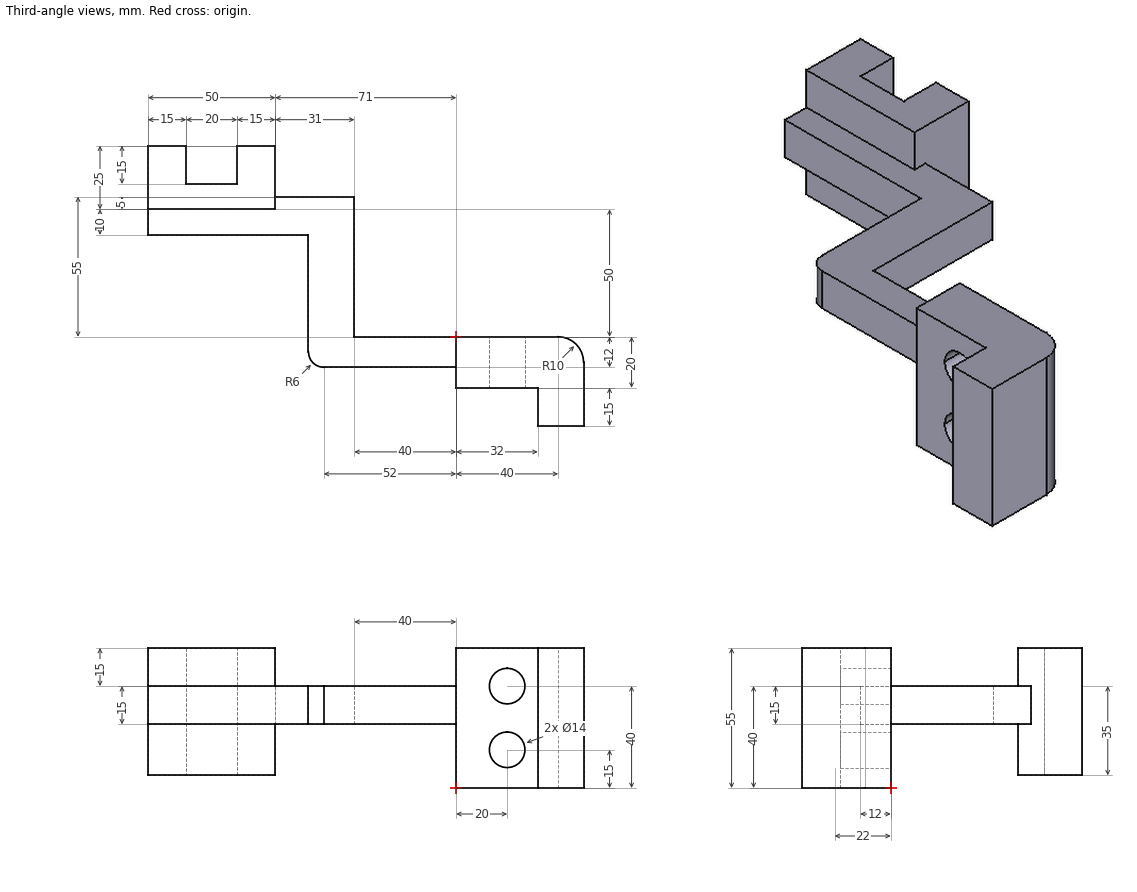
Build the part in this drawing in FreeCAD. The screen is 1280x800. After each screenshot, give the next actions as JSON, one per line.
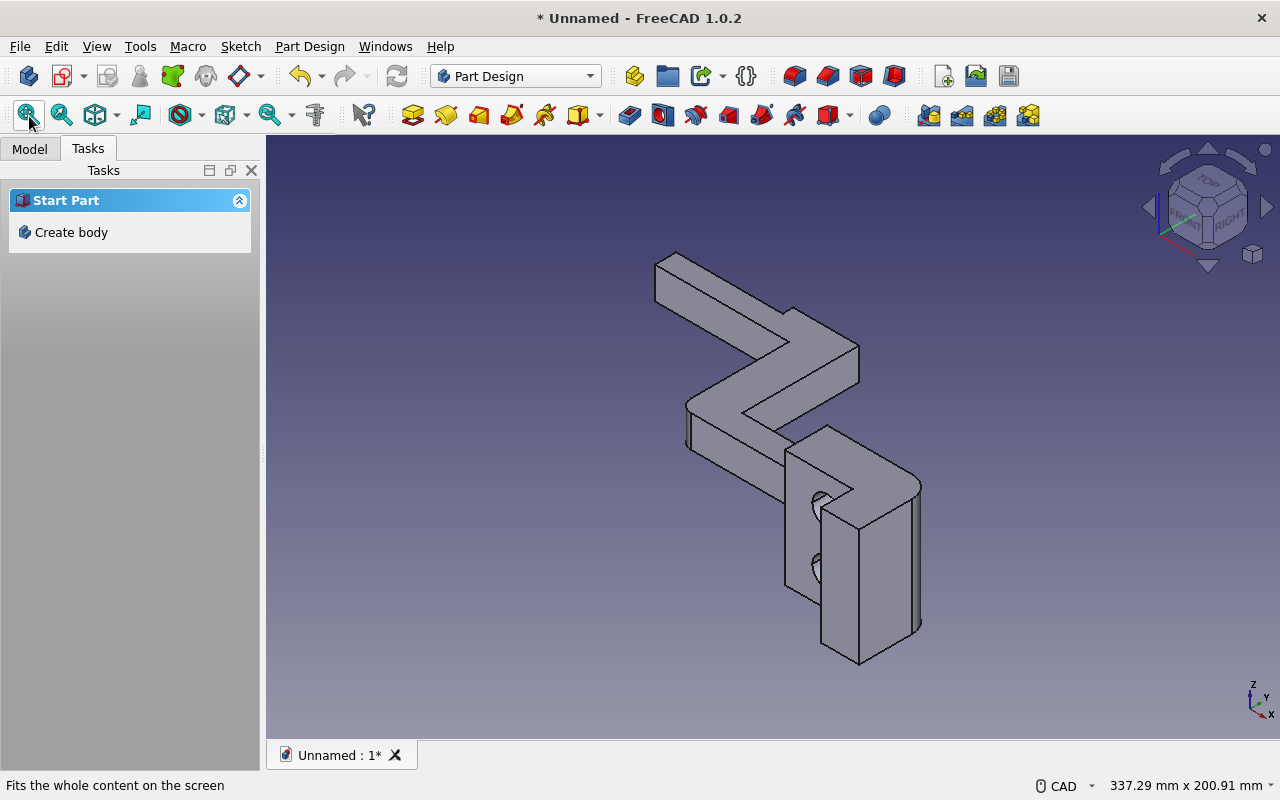
{"action": "left_click", "coordinate": [757, 438]}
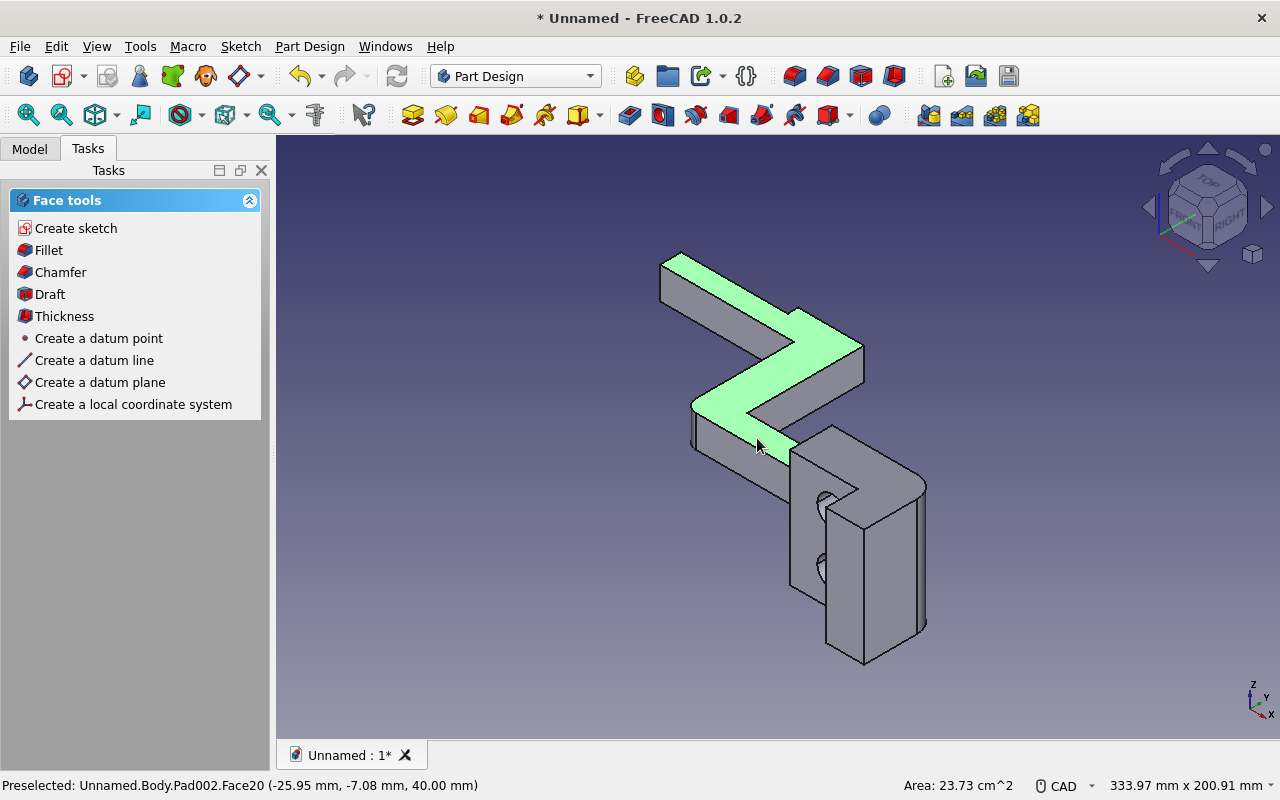
{"action": "left_click", "coordinate": [62, 76]}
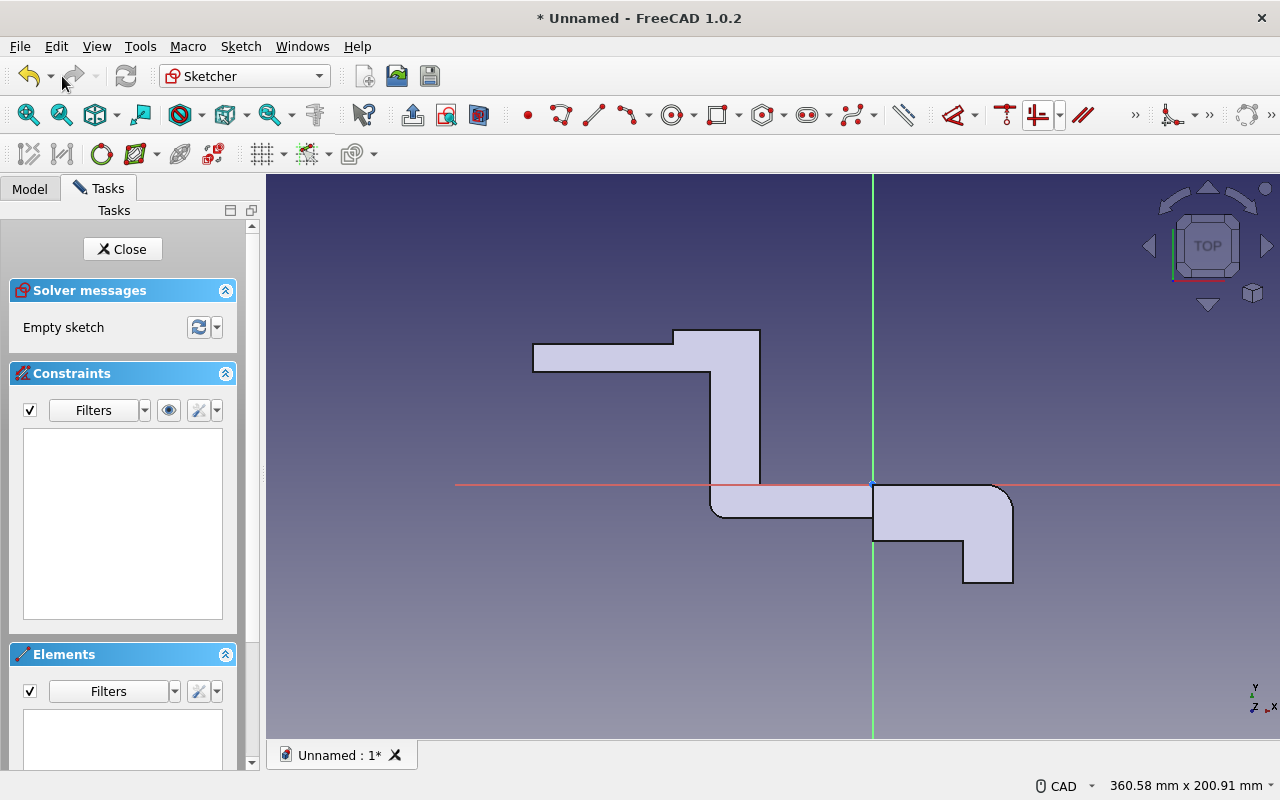
{"action": "left_click", "coordinate": [479, 116]}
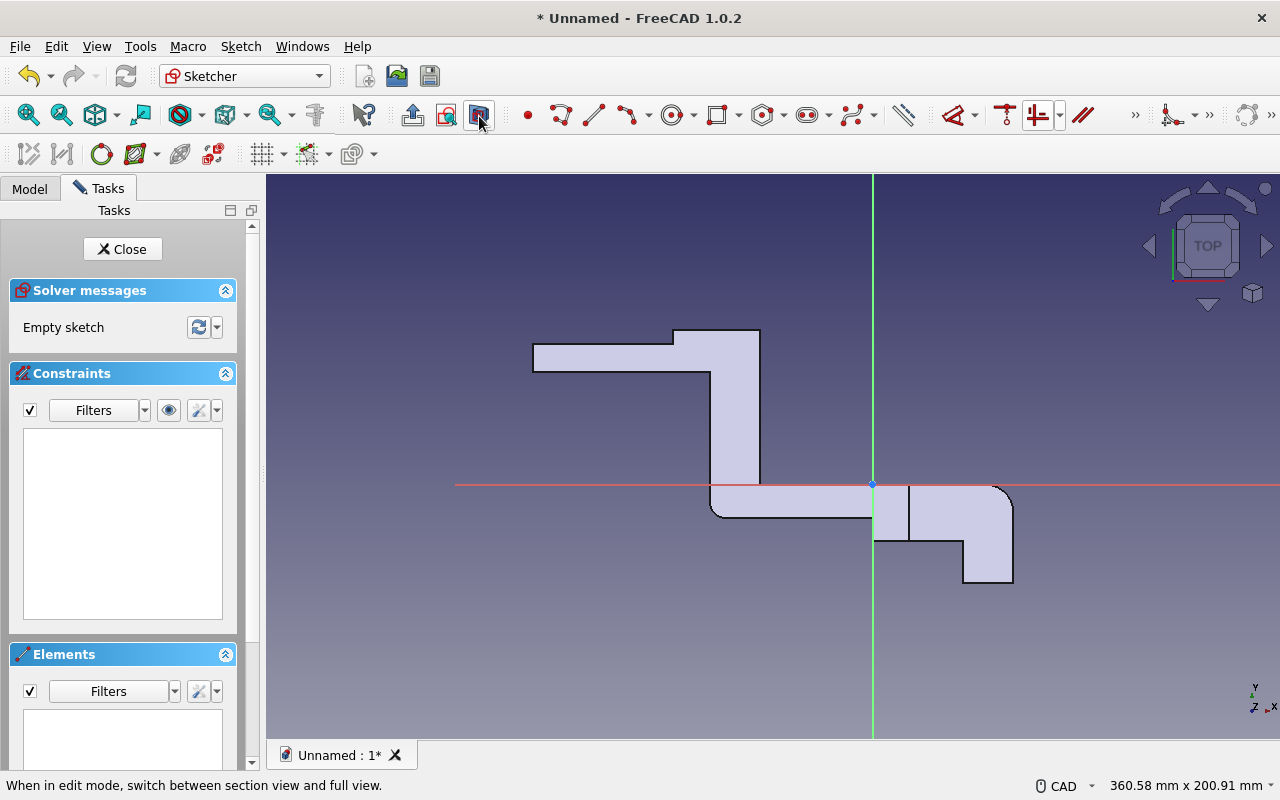
{"action": "scroll", "coordinate": [701, 285], "scroll_direction": "up", "scroll_amount": 3}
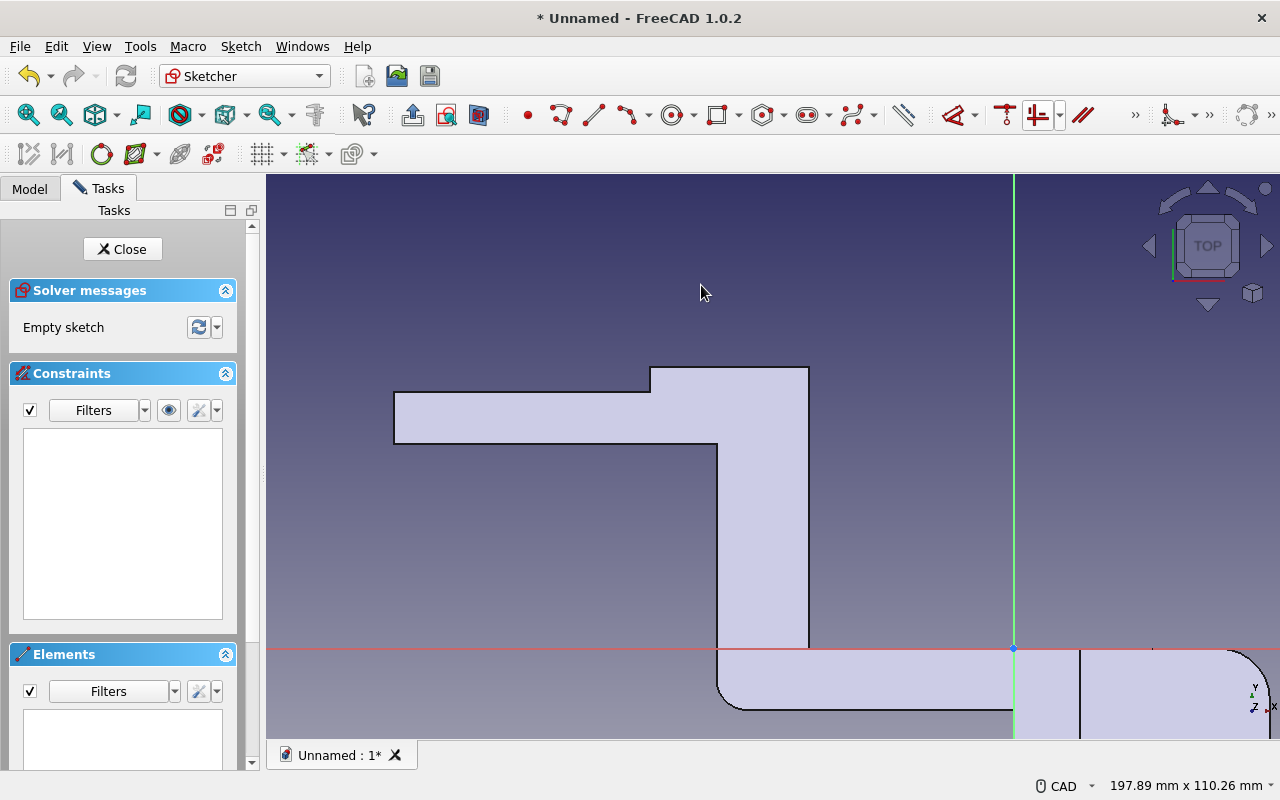
{"action": "left_click", "coordinate": [561, 116]}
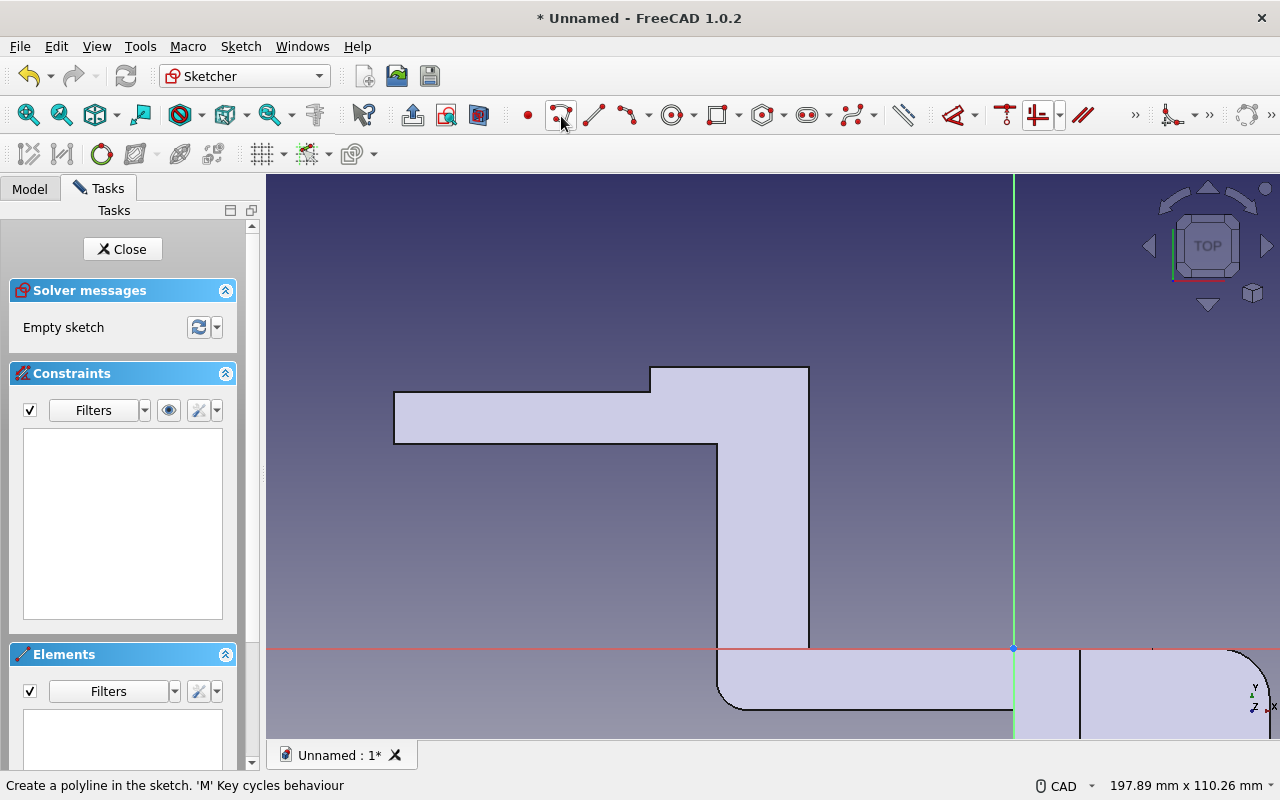
{"action": "left_click", "coordinate": [650, 392]}
{"action": "left_click", "coordinate": [650, 264]}
{"action": "left_click", "coordinate": [573, 264]}
{"action": "left_click", "coordinate": [573, 341]}
{"action": "left_click", "coordinate": [471, 341]}
{"action": "left_click", "coordinate": [471, 264]}
{"action": "left_click", "coordinate": [394, 264]}
{"action": "left_click", "coordinate": [394, 392]}
{"action": "left_click", "coordinate": [650, 393]}
{"action": "key", "text": "Escape"}
{"action": "key", "text": "Escape"}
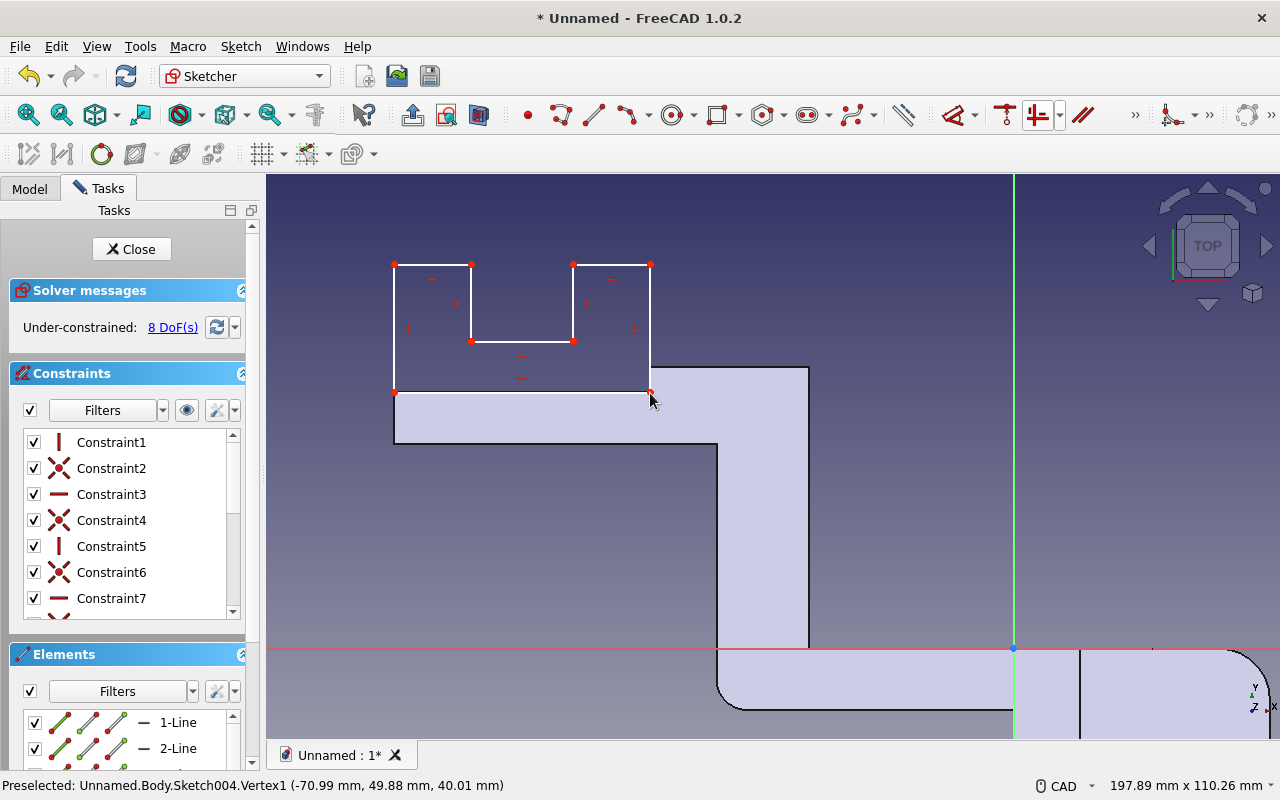
{"action": "left_click", "coordinate": [952, 116]}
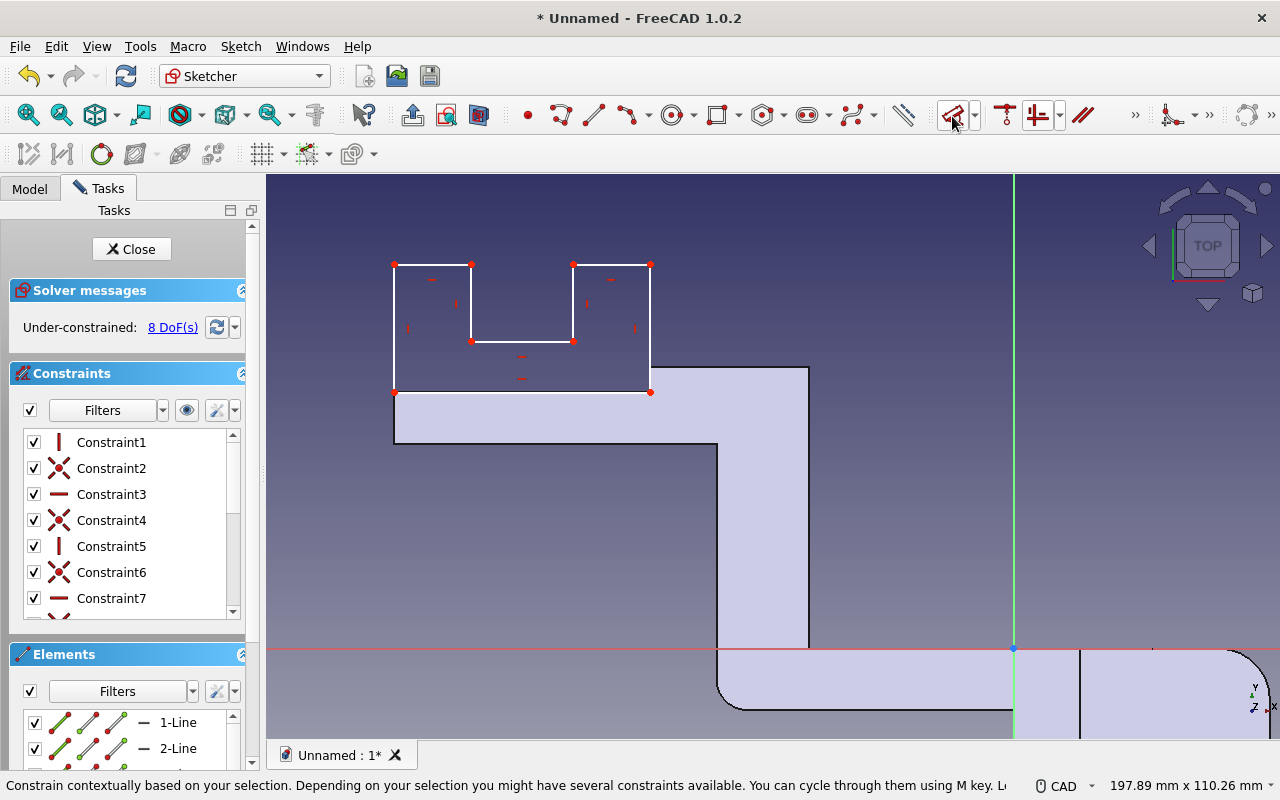
{"action": "left_click", "coordinate": [650, 355]}
{"action": "left_click", "coordinate": [616, 329]}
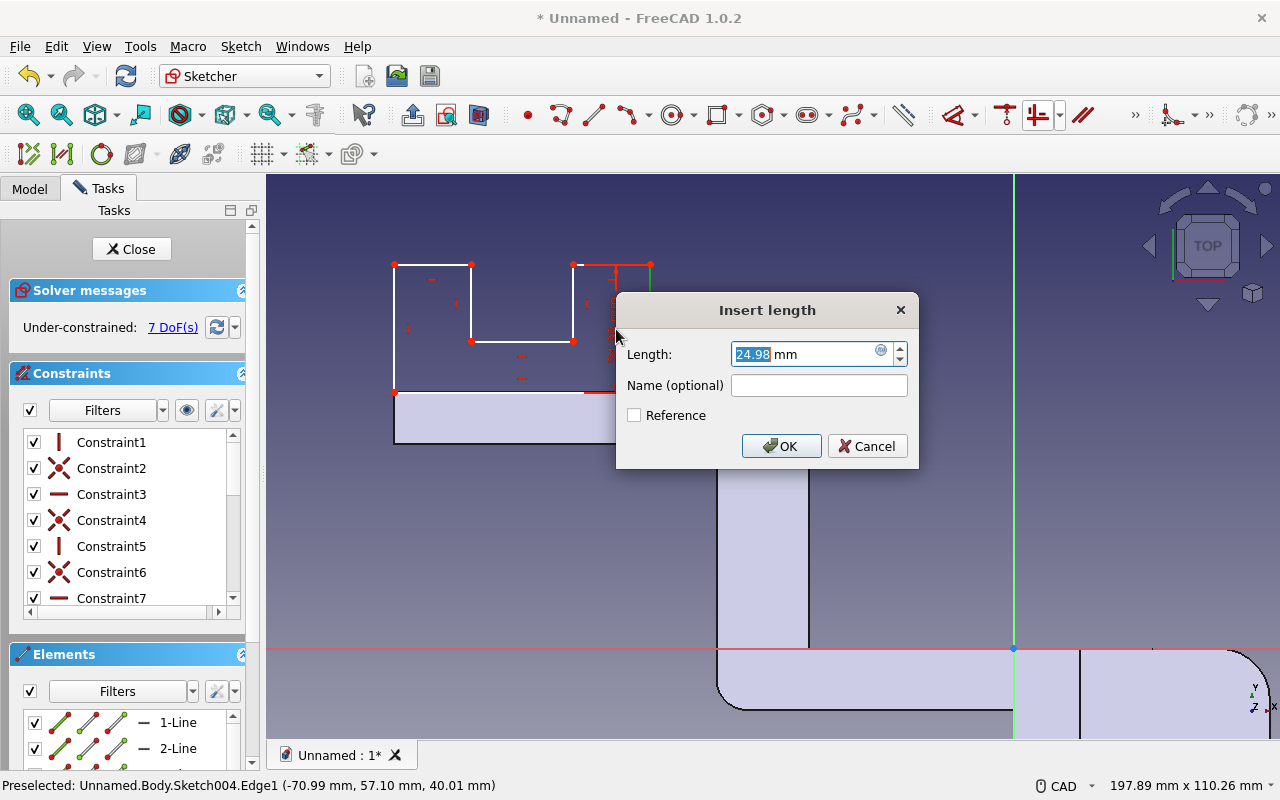
{"action": "type", "text": "25"}
{"action": "key", "text": "Return"}